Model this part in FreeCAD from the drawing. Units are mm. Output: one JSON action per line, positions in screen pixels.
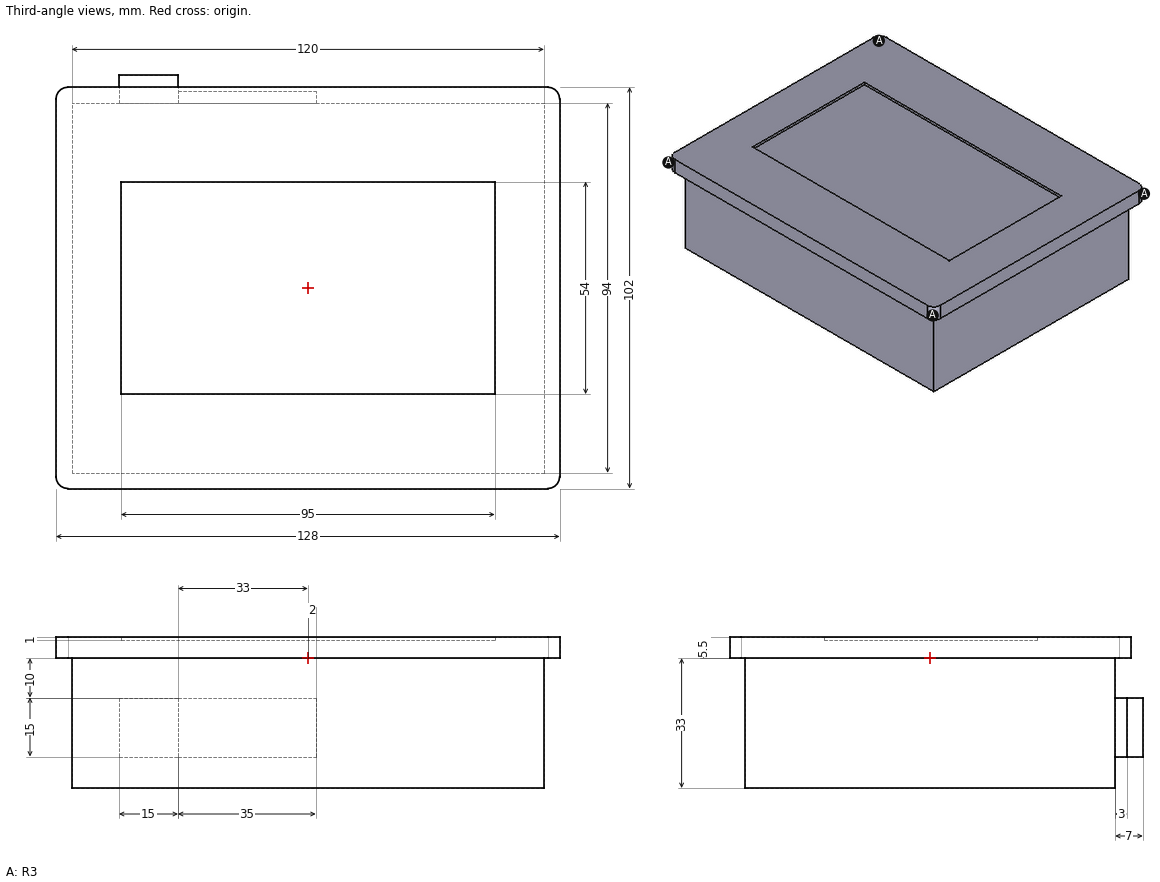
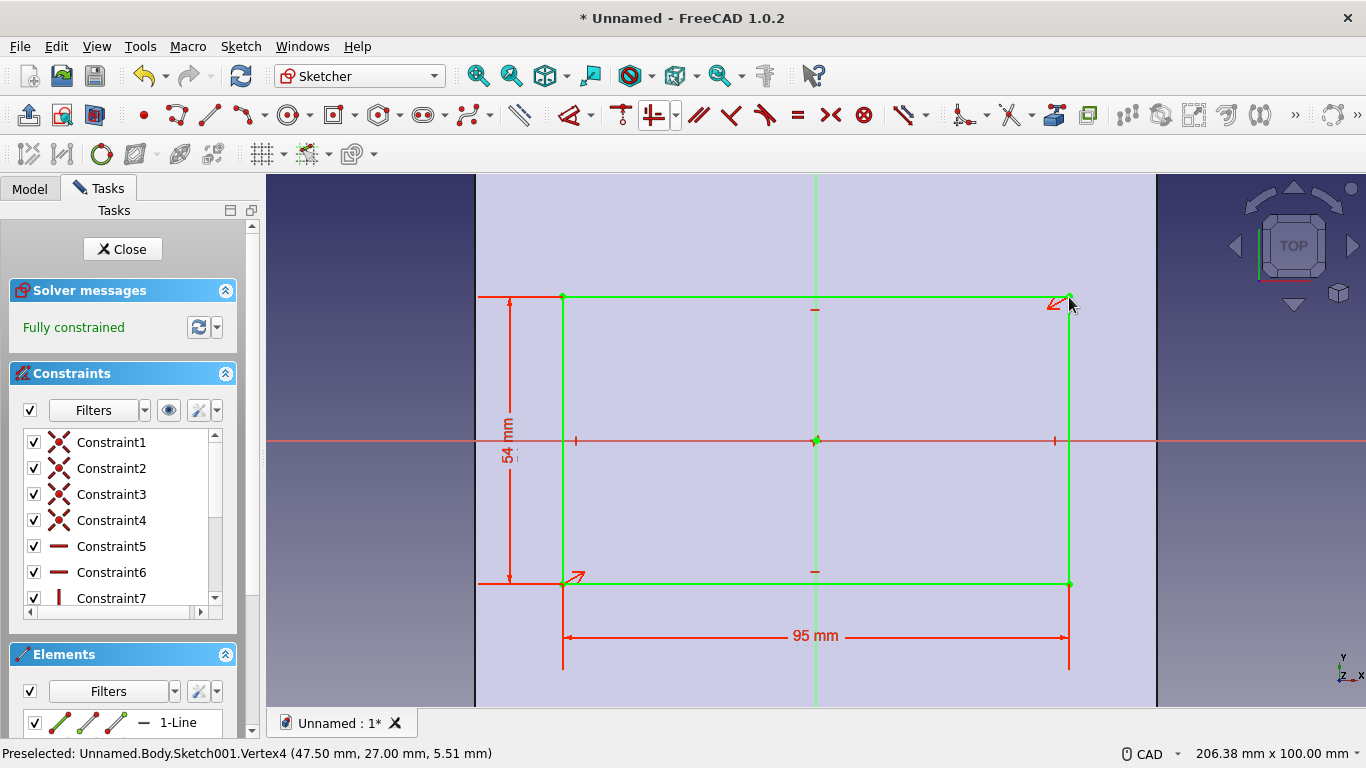
{"action": "left_click", "coordinate": [123, 249]}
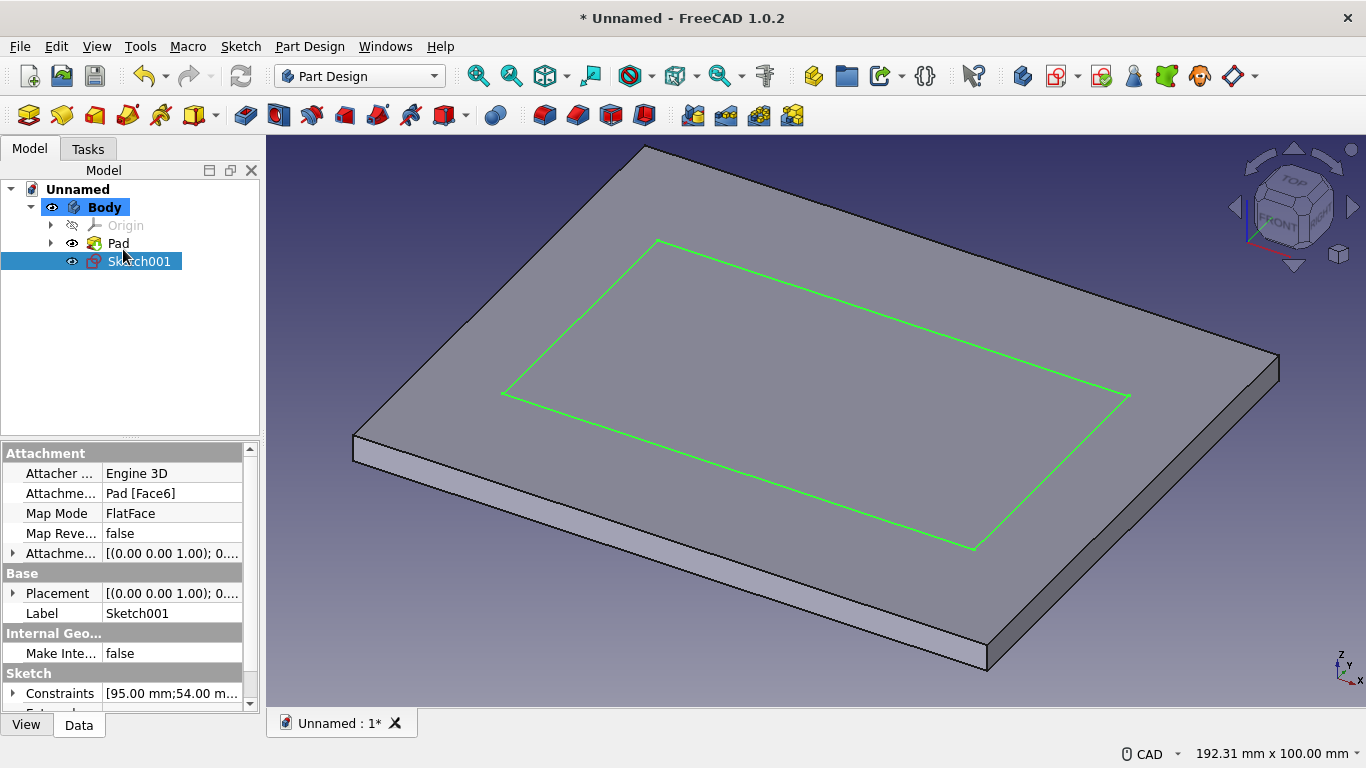
{"action": "left_click", "coordinate": [246, 116]}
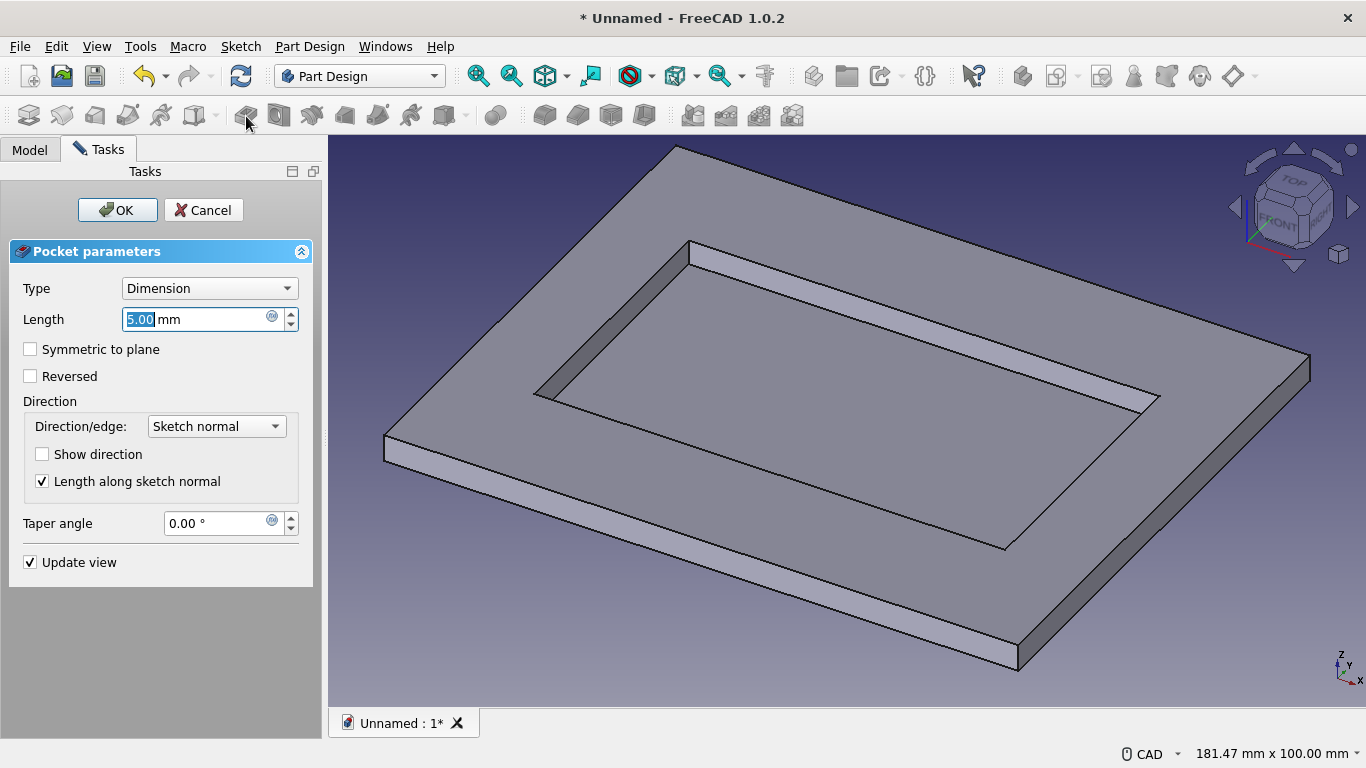
{"action": "type", "text": "1"}
{"action": "key", "text": "Tab"}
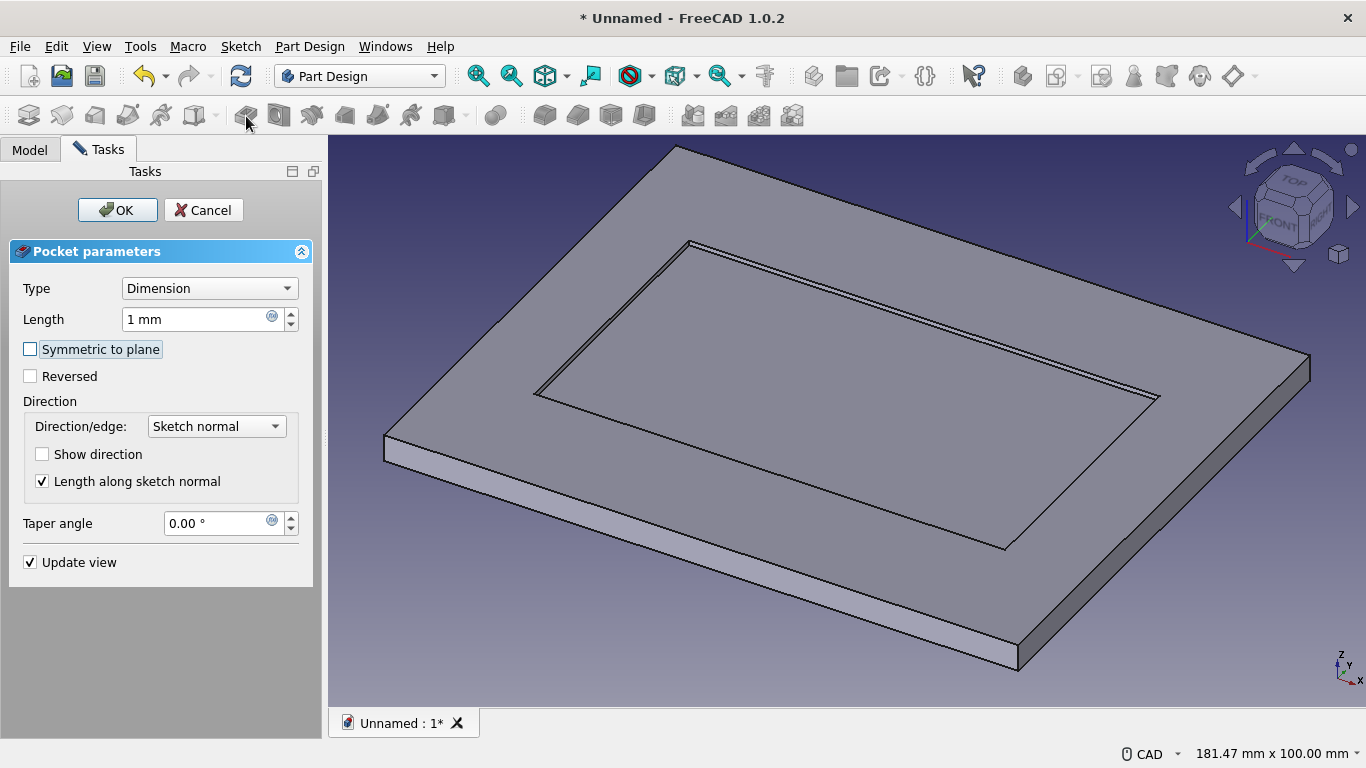
{"action": "left_click", "coordinate": [118, 210]}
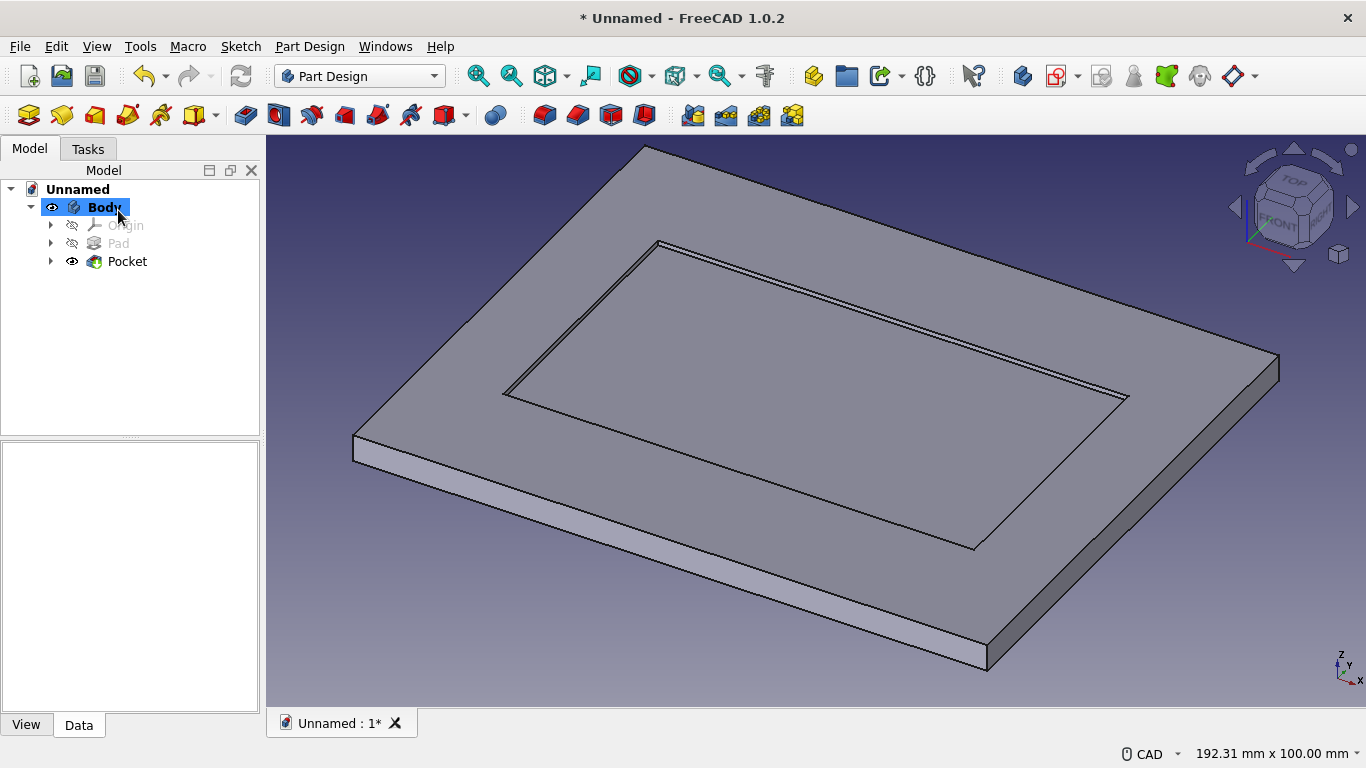
{"action": "key", "text": "5"}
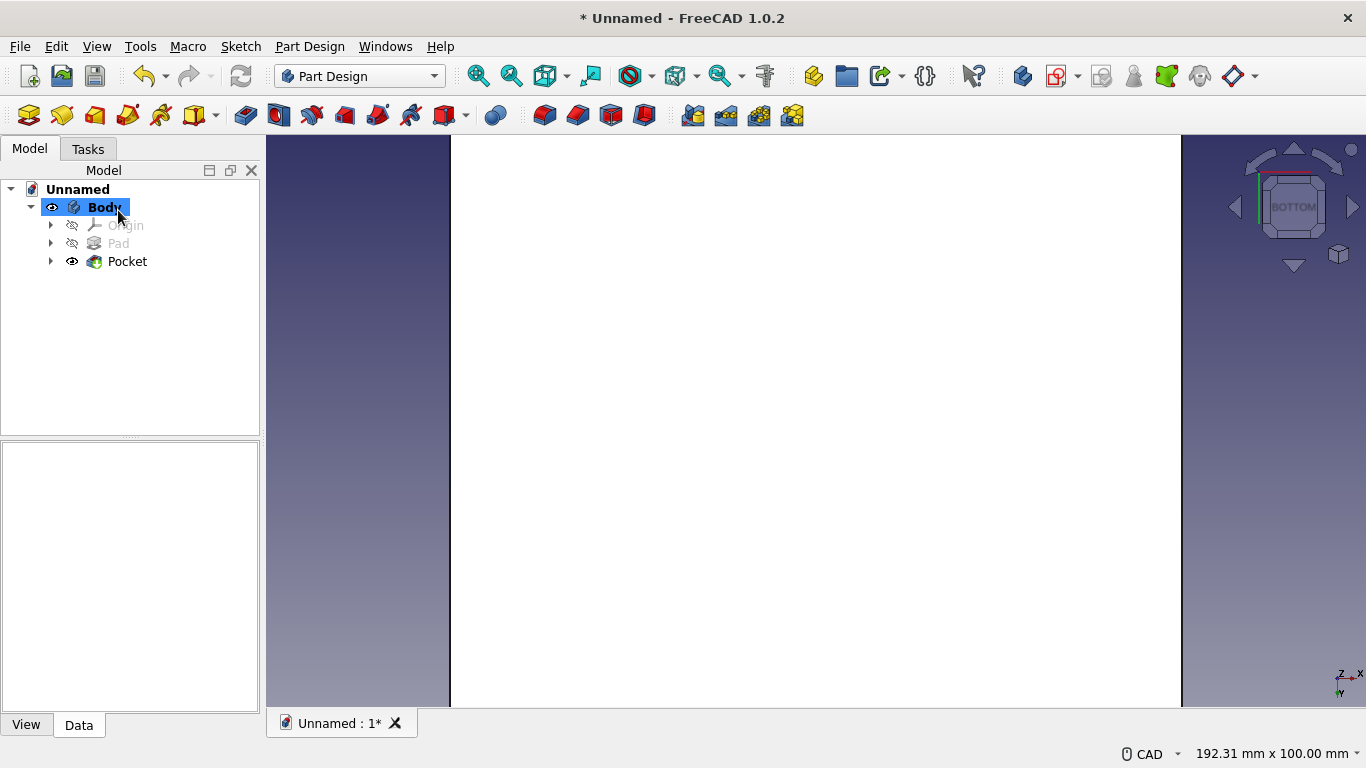
{"action": "left_click", "coordinate": [479, 76]}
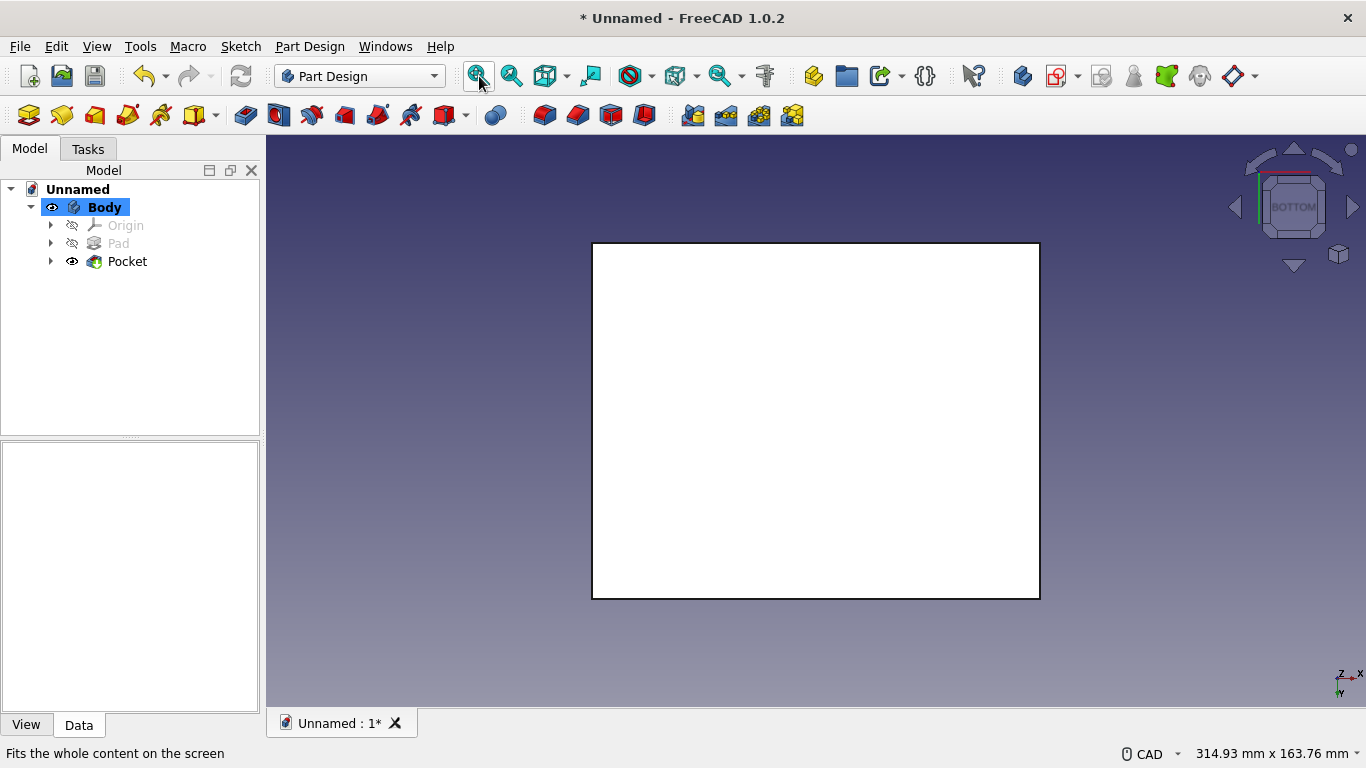
{"action": "left_click", "coordinate": [816, 420]}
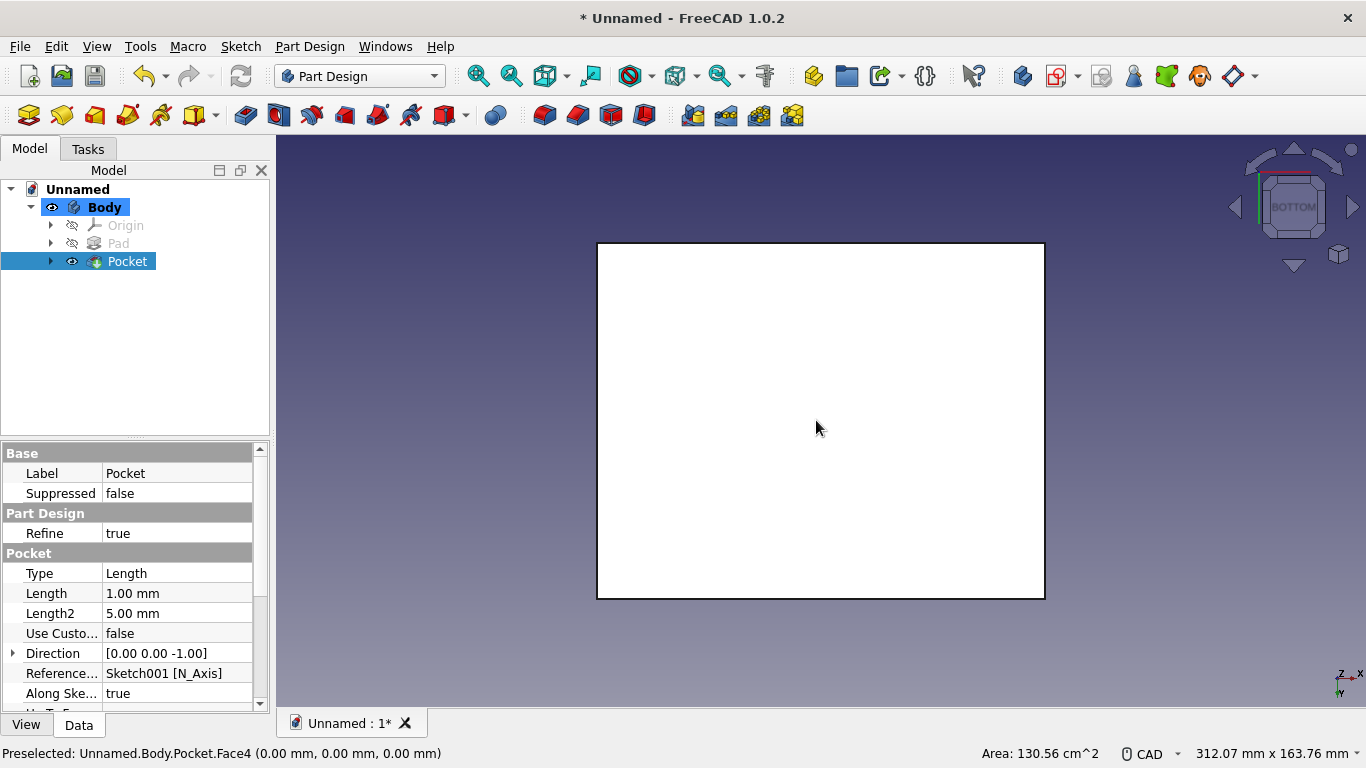
{"action": "left_click", "coordinate": [1056, 76]}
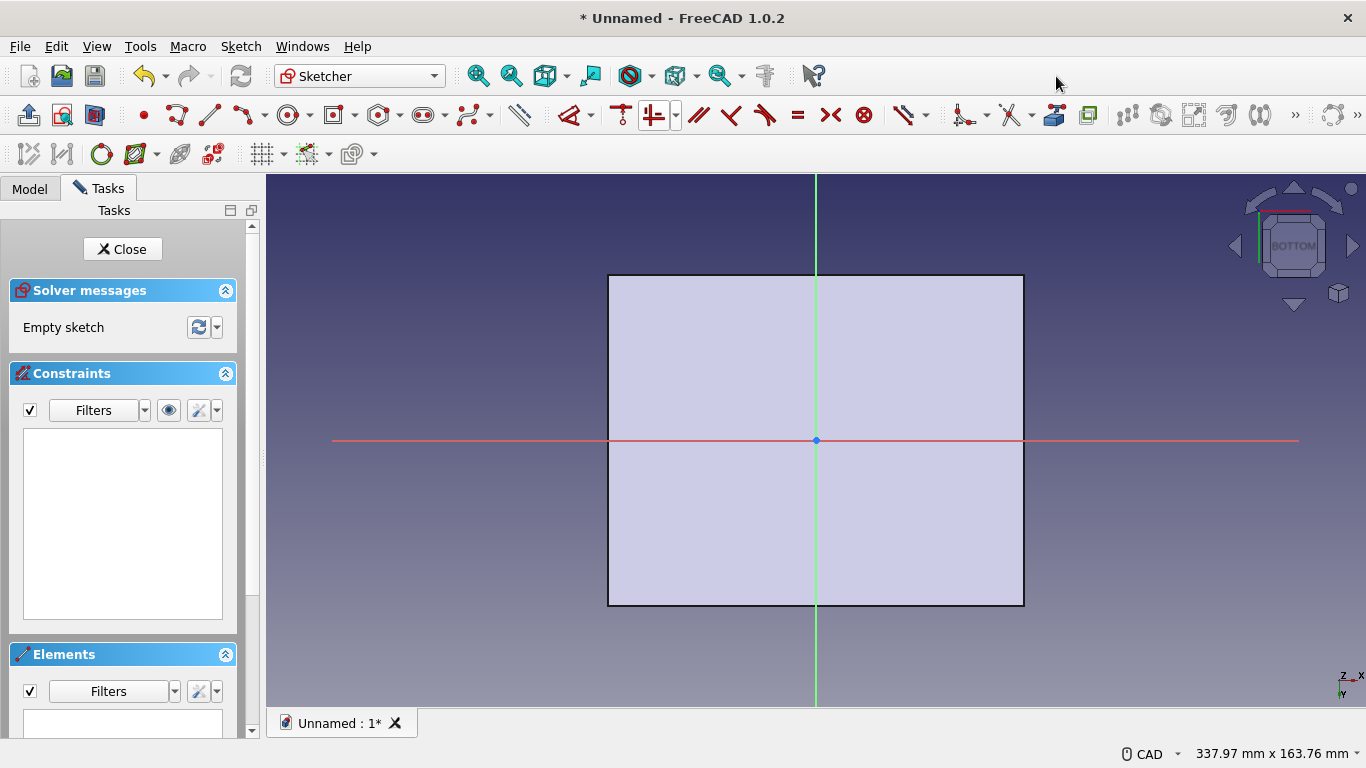
{"action": "key", "text": "g v"}